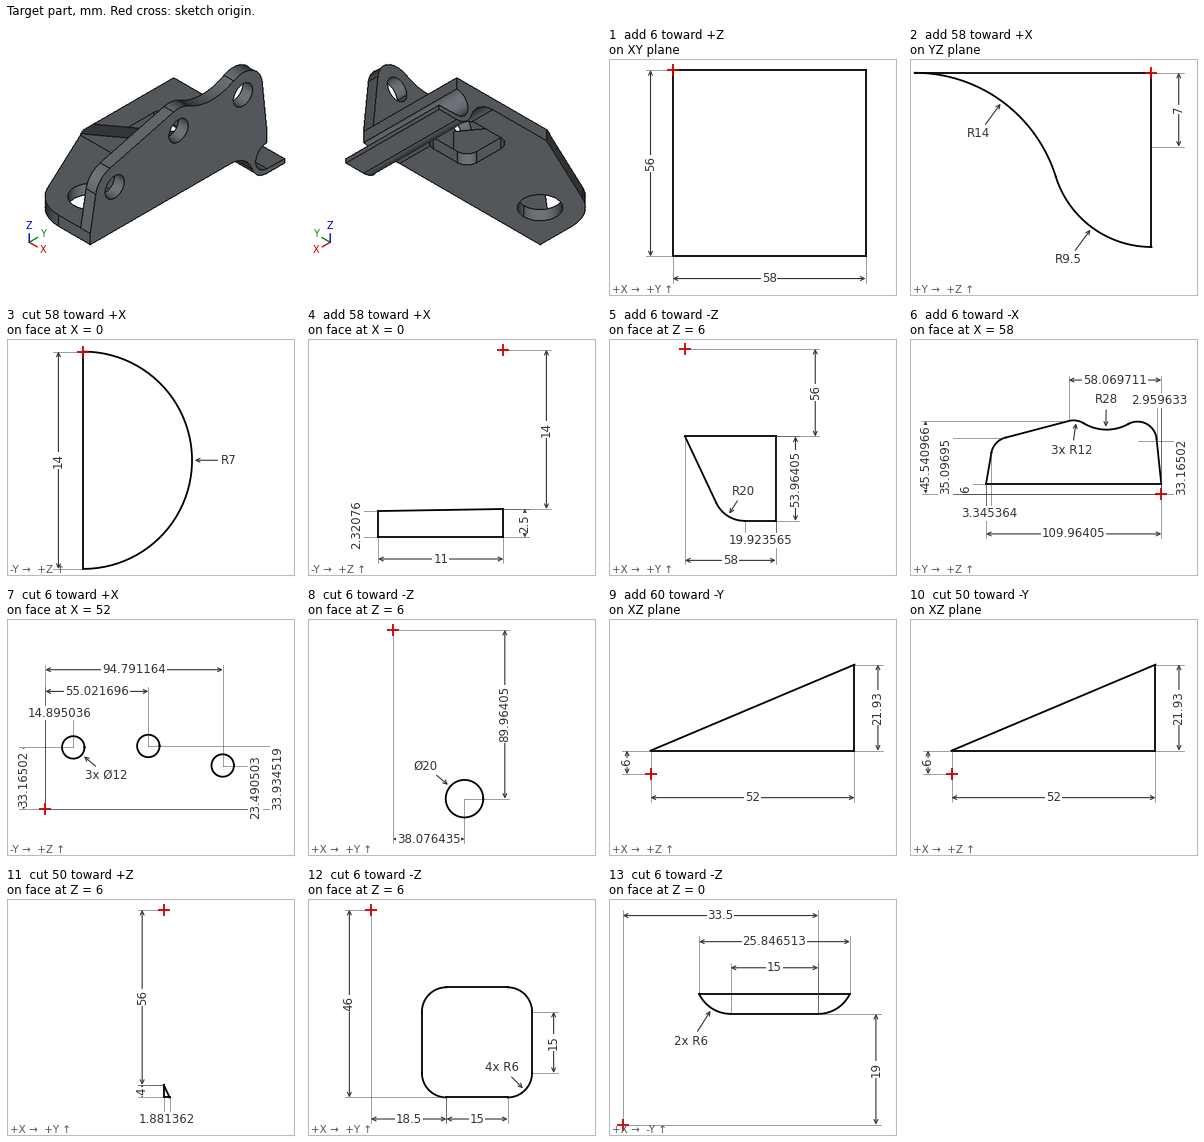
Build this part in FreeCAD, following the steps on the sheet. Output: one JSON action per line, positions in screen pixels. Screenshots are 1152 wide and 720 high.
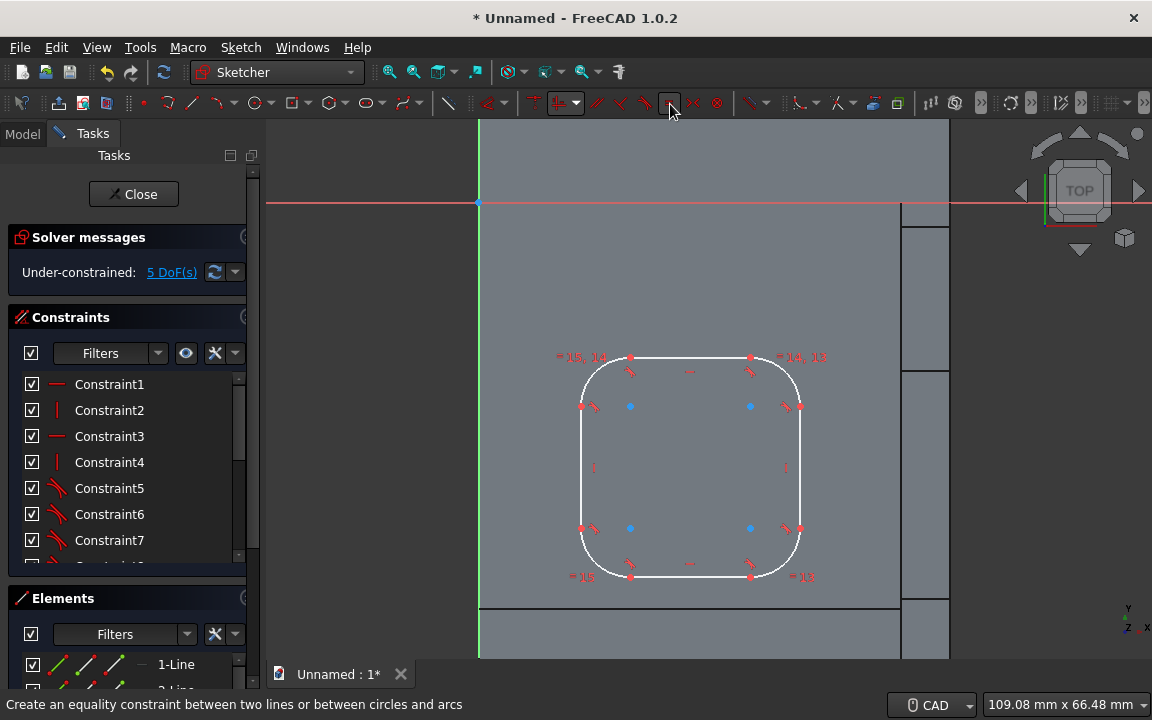
{"action": "key", "text": "d"}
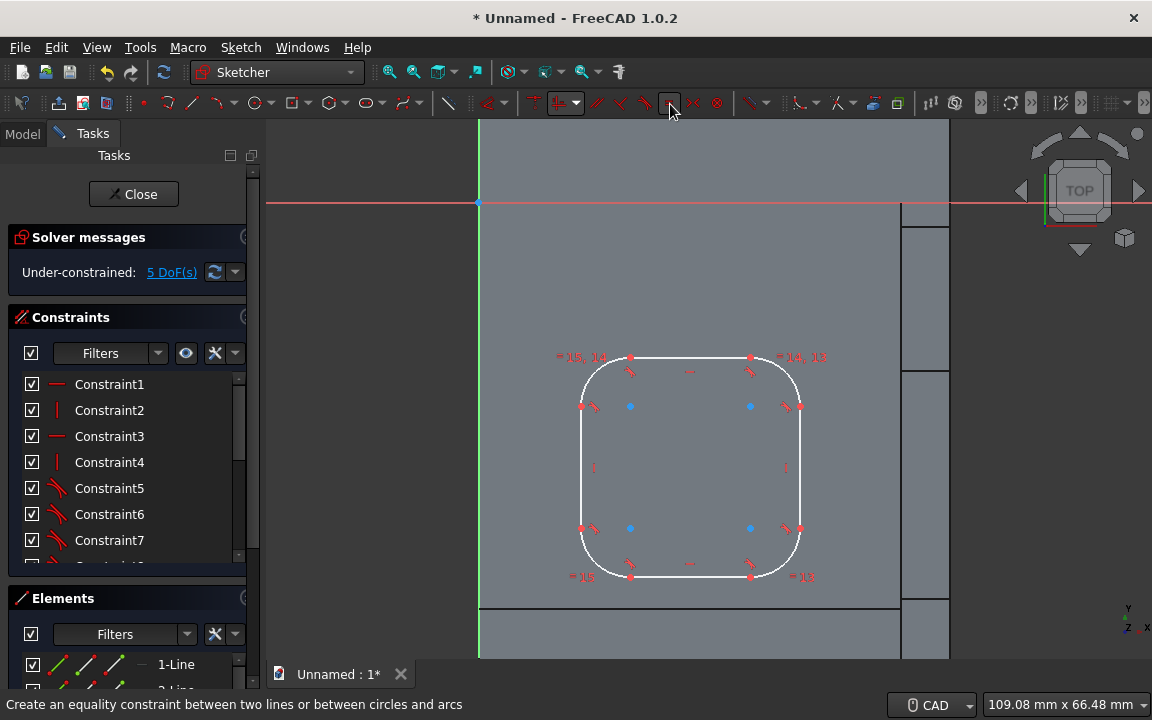
{"action": "left_click", "coordinate": [773, 572]}
{"action": "left_click", "coordinate": [787, 601]}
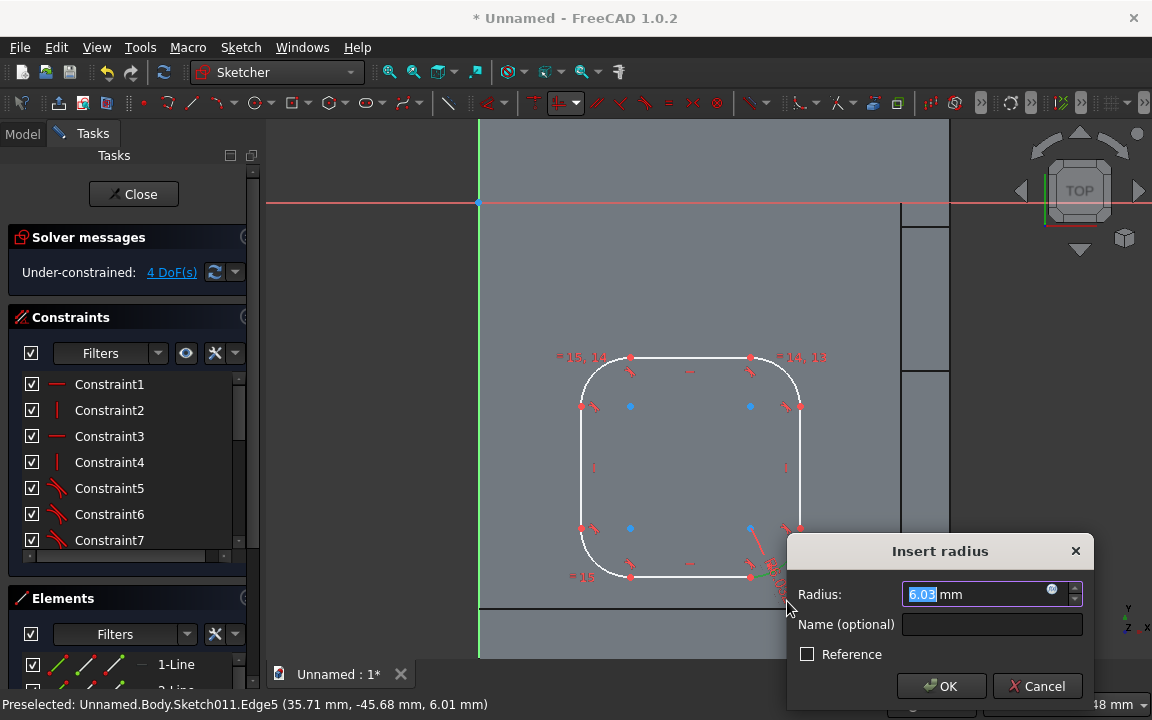
{"action": "type", "text": "6"}
{"action": "key", "text": "Return"}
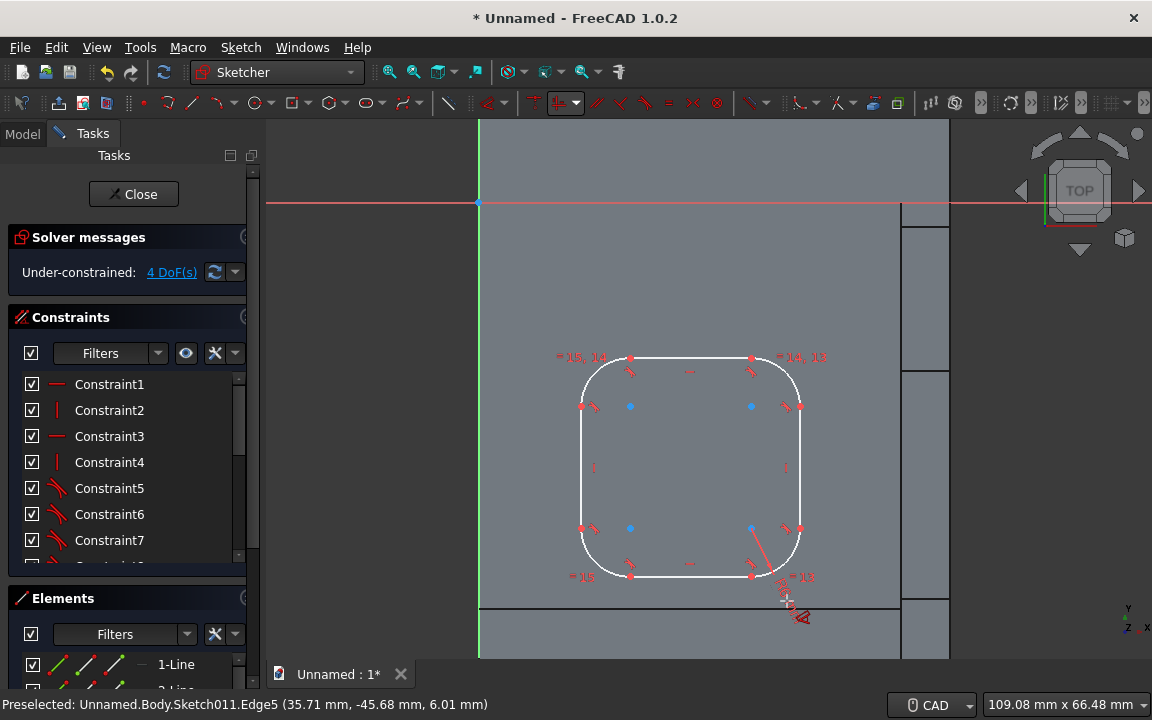
{"action": "left_click", "coordinate": [666, 577]}
{"action": "left_click", "coordinate": [691, 611]}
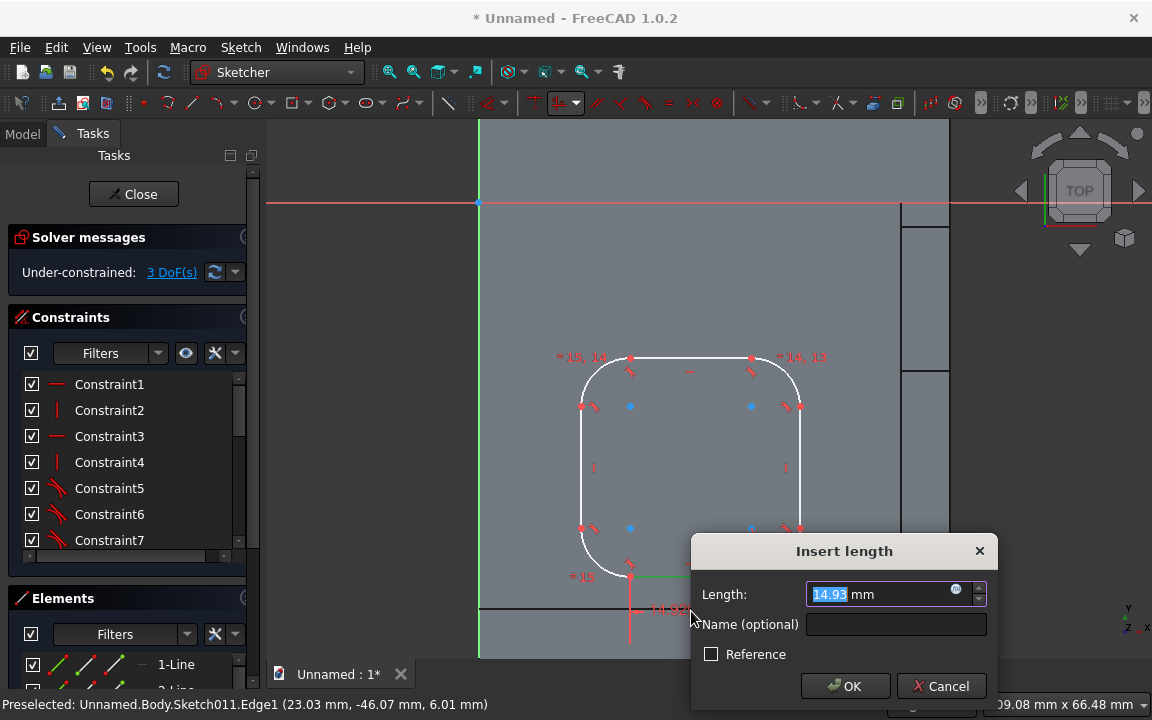
{"action": "type", "text": "15"}
{"action": "key", "text": "Return"}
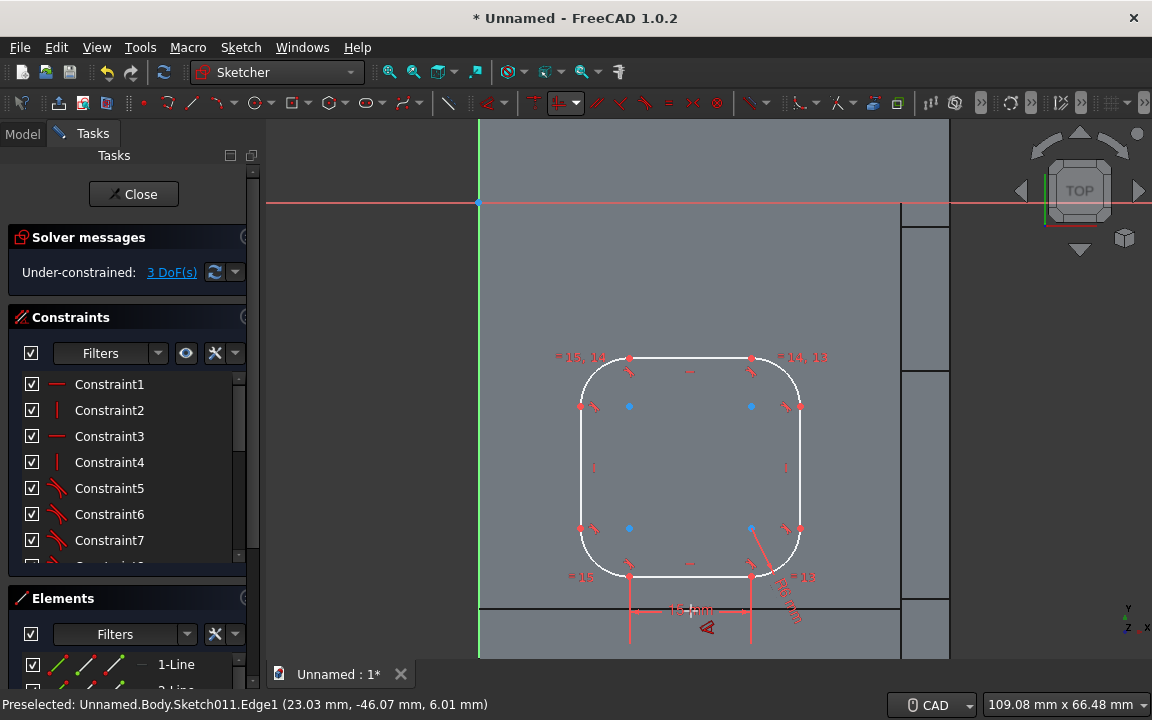
{"action": "left_click", "coordinate": [800, 492]}
{"action": "left_click", "coordinate": [834, 467]}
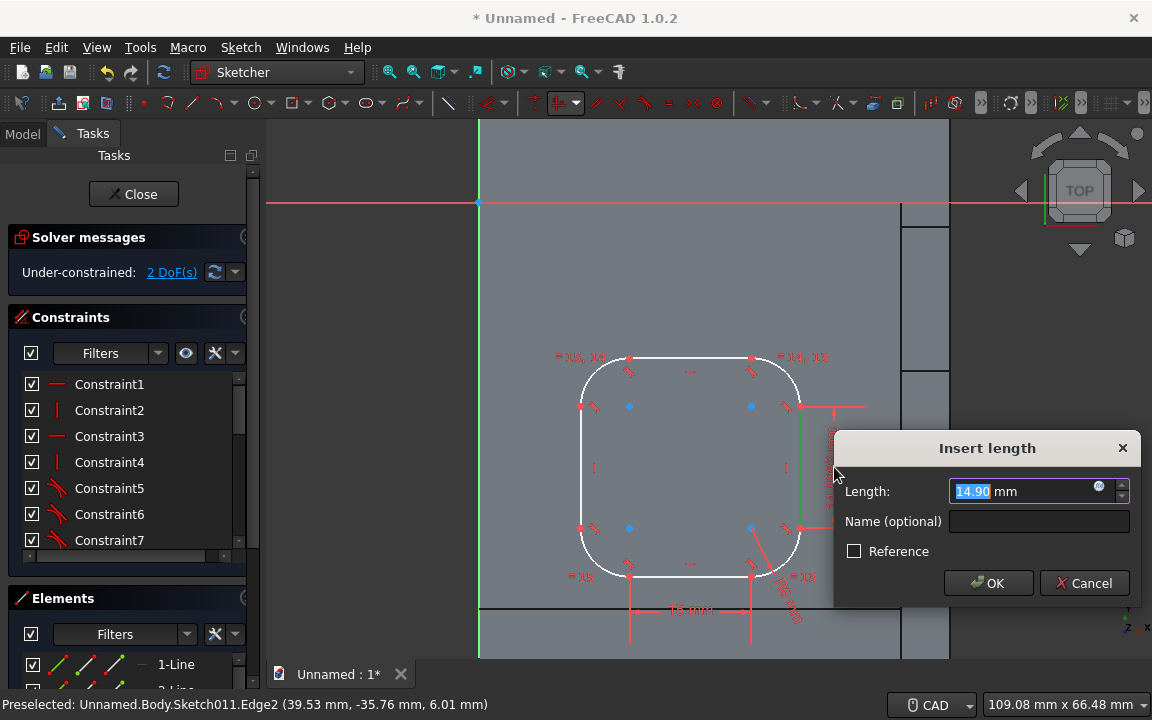
{"action": "type", "text": "15"}
{"action": "key", "text": "Return"}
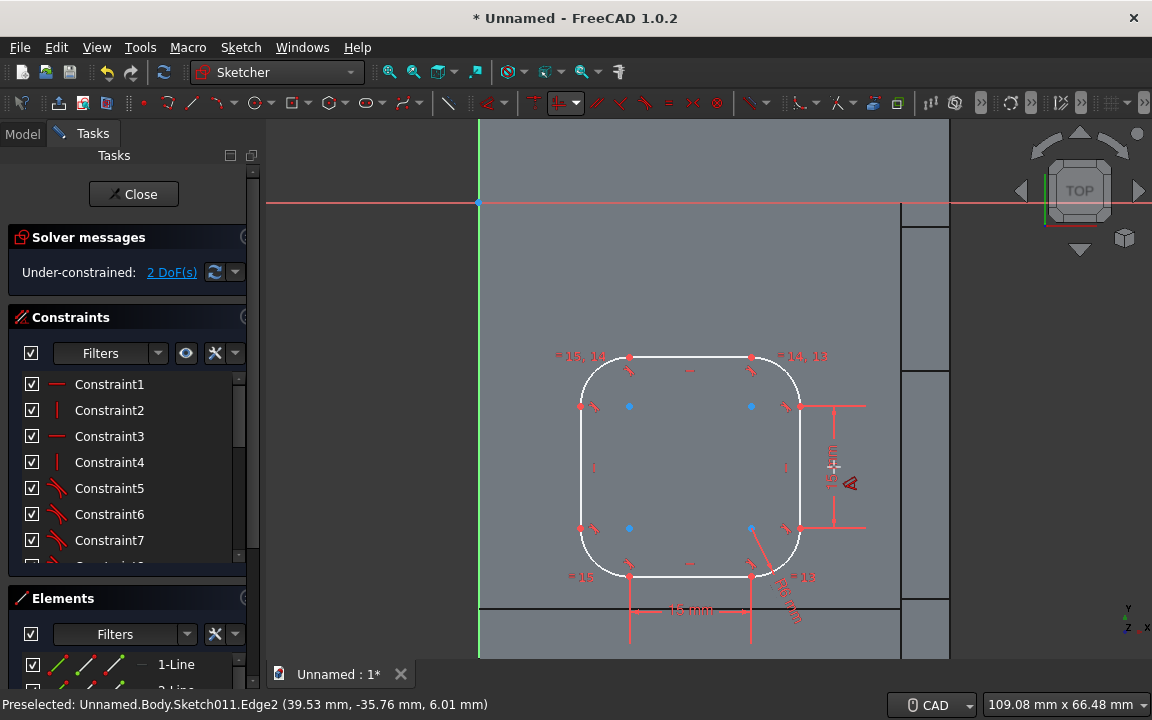
{"action": "left_click", "coordinate": [630, 577]}
{"action": "left_click", "coordinate": [445, 390]}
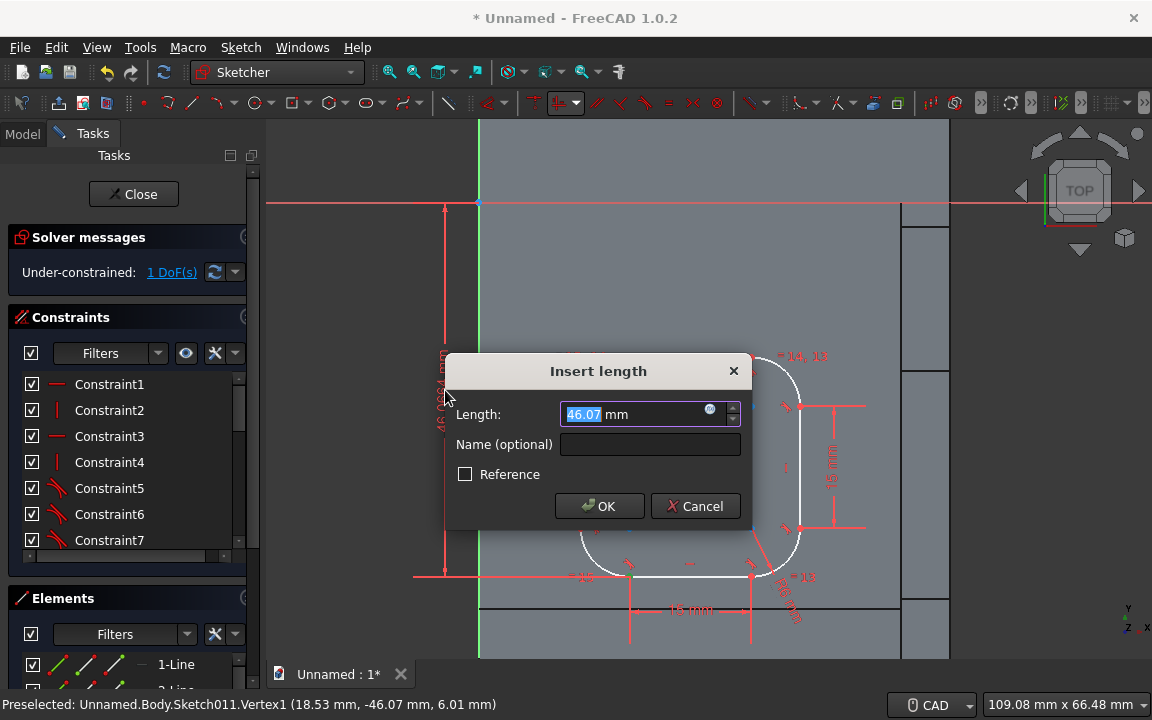
{"action": "type", "text": "46"}
{"action": "key", "text": "Return"}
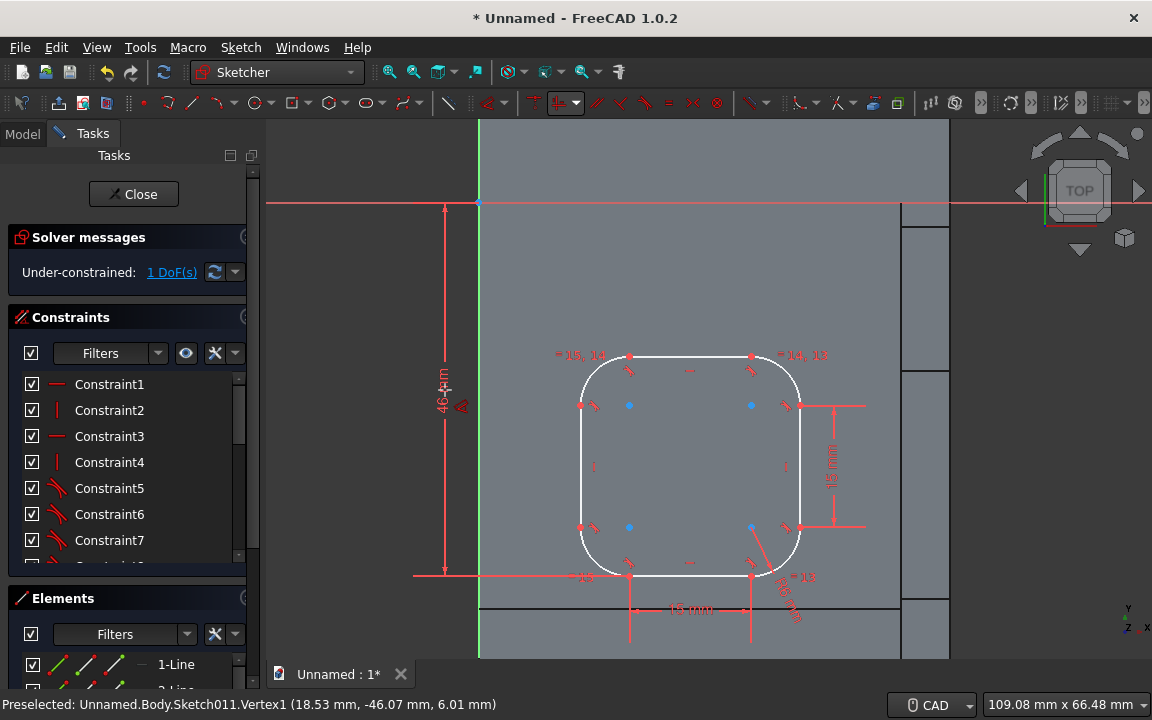
{"action": "left_click", "coordinate": [630, 576]}
{"action": "left_click", "coordinate": [554, 610]}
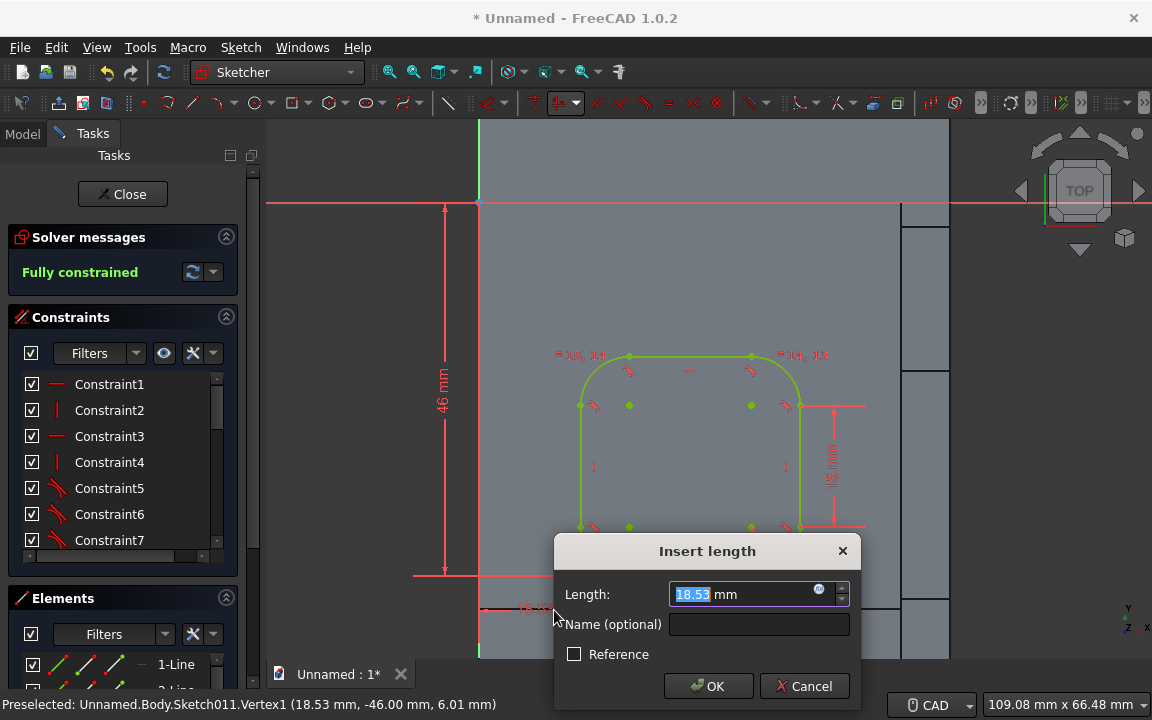
{"action": "type", "text": "18.5"}
{"action": "key", "text": "Return"}
{"action": "key", "text": "Escape"}